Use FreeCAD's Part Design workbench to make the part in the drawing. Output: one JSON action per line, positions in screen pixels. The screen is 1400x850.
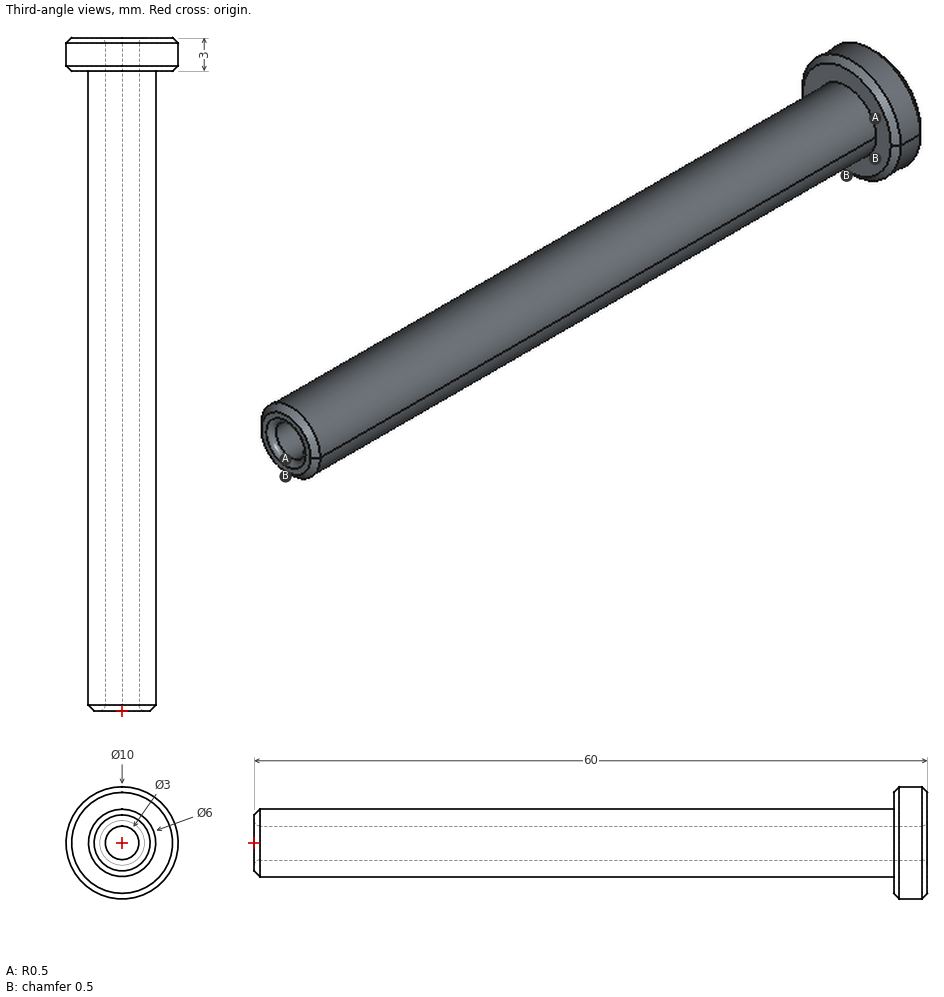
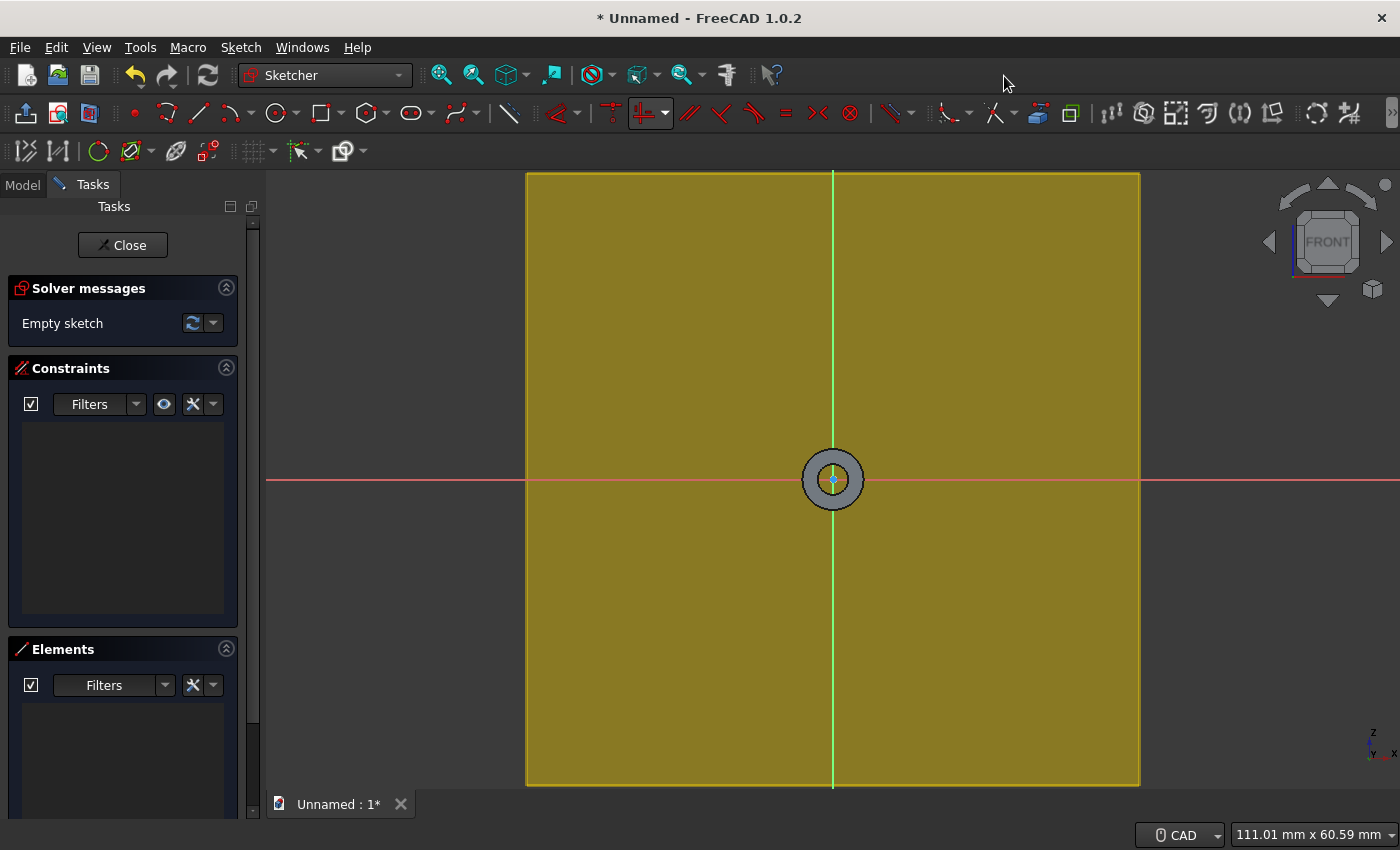
{"action": "left_click", "coordinate": [90, 114]}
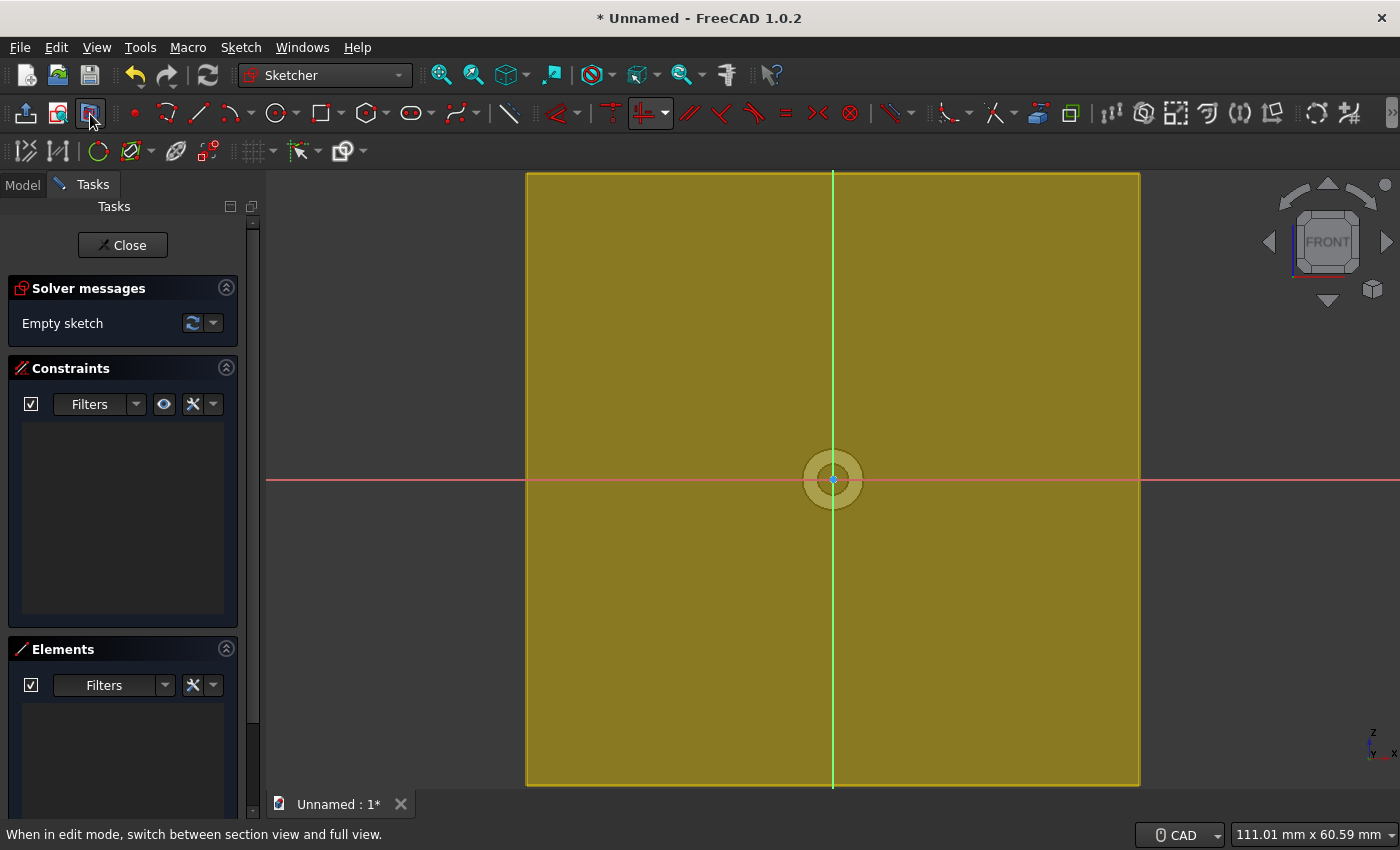
{"action": "scroll", "coordinate": [855, 480], "scroll_direction": "up", "scroll_amount": 7}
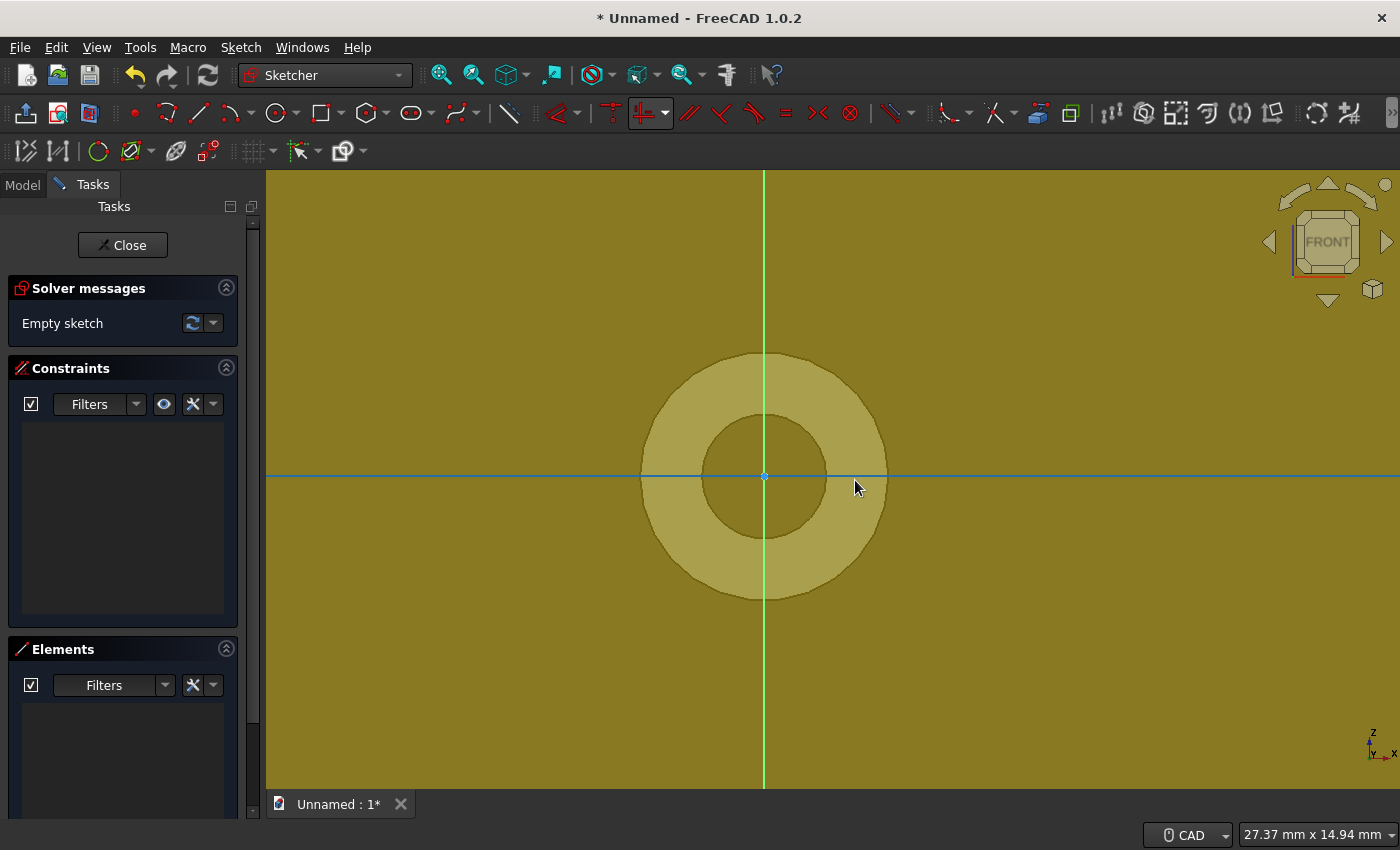
{"action": "key", "text": "g c"}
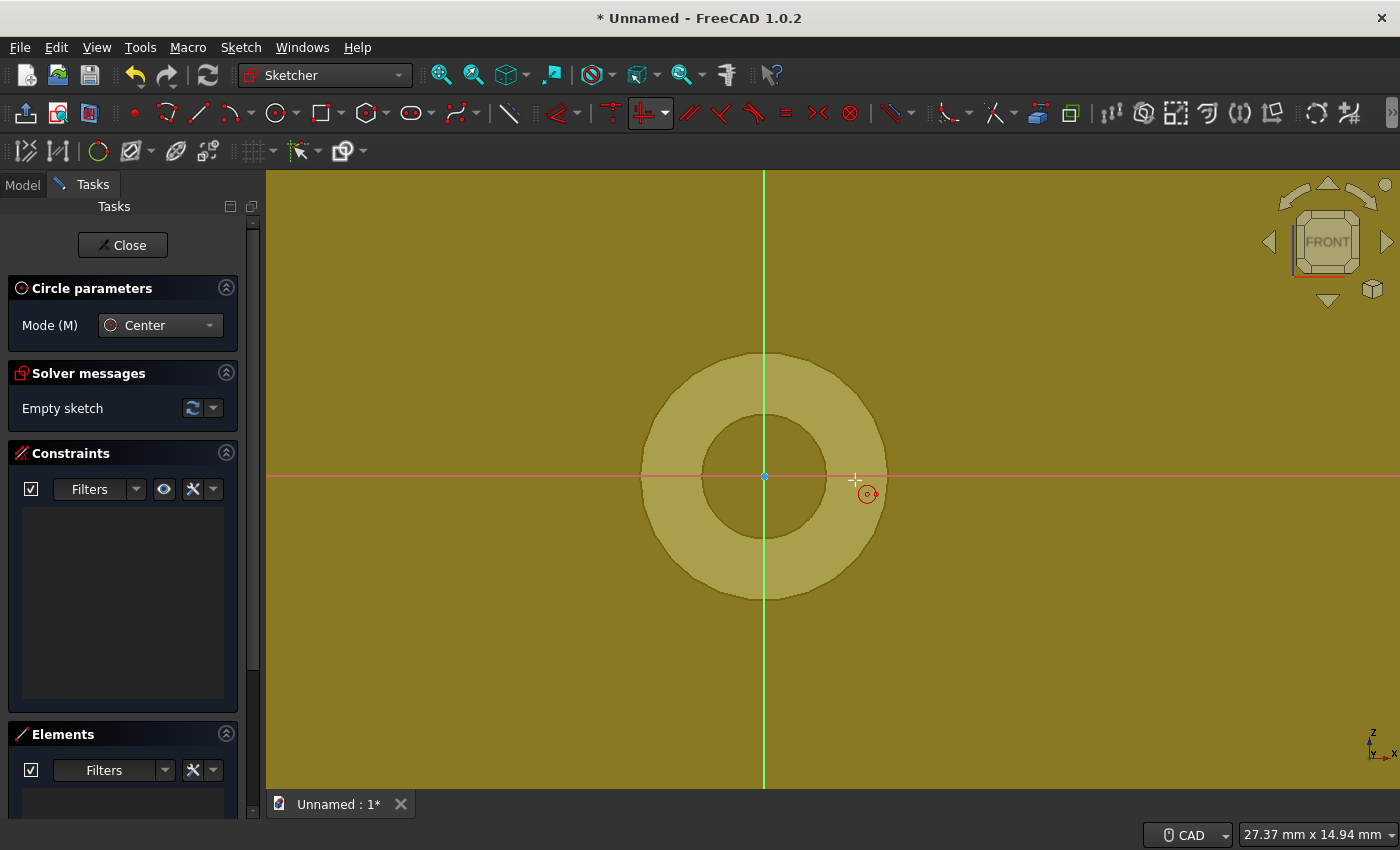
{"action": "left_click", "coordinate": [764, 476]}
{"action": "mouse_move", "coordinate": [911, 330]}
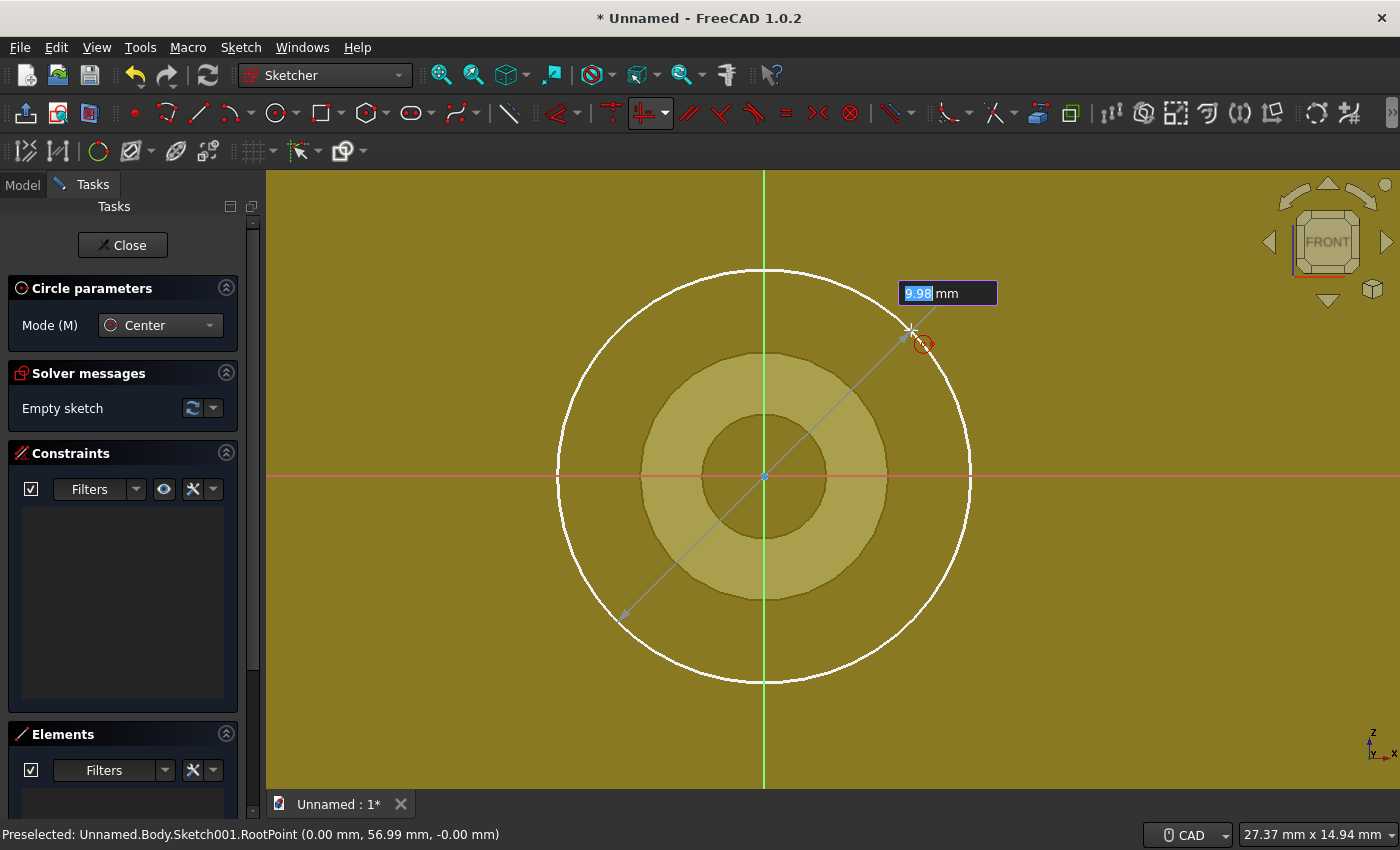
{"action": "type", "text": "10"}
{"action": "key", "text": "Return"}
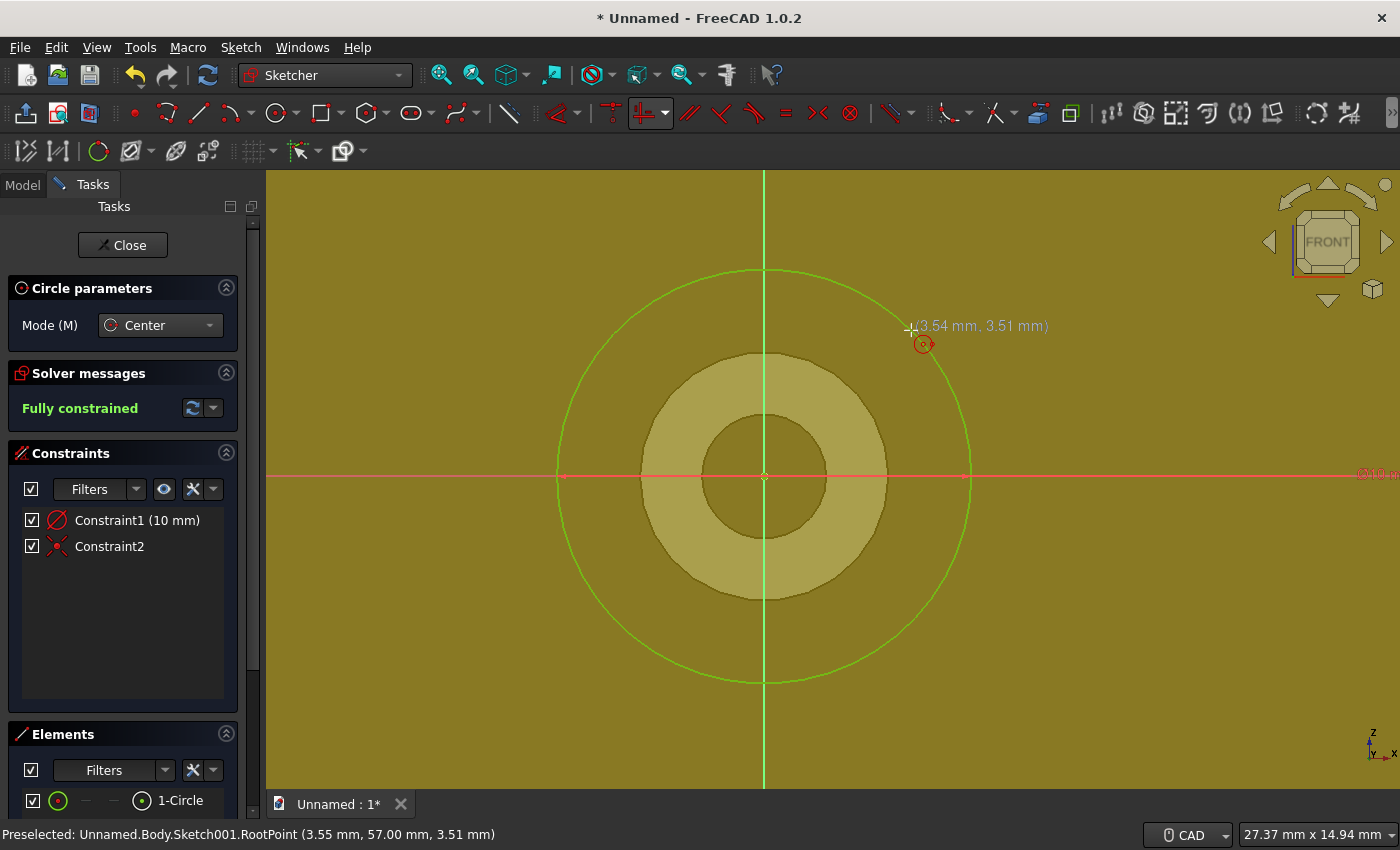
{"action": "left_click", "coordinate": [764, 476]}
{"action": "mouse_move", "coordinate": [808, 433]}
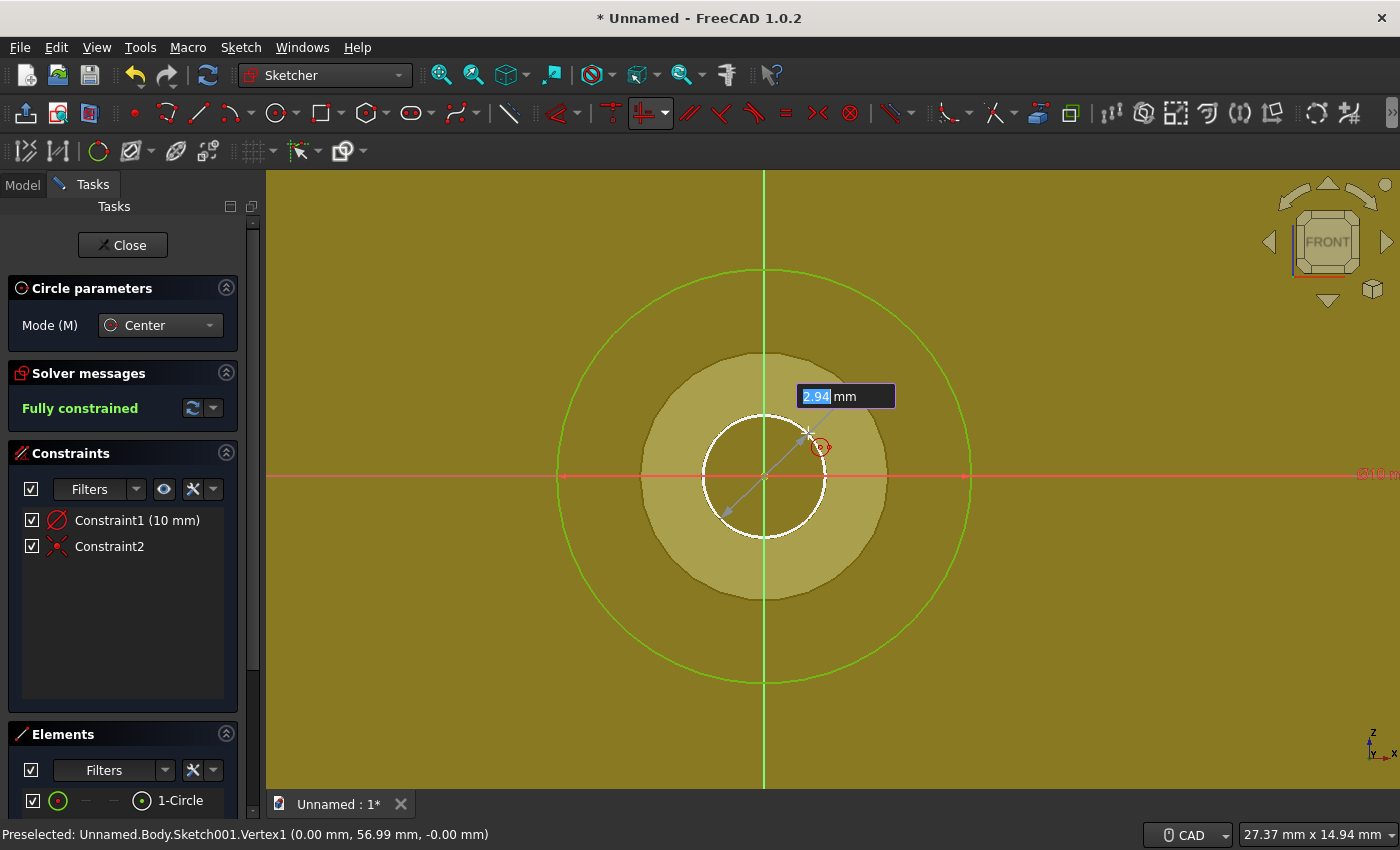
{"action": "type", "text": "3"}
{"action": "key", "text": "Return"}
{"action": "key", "text": "Escape"}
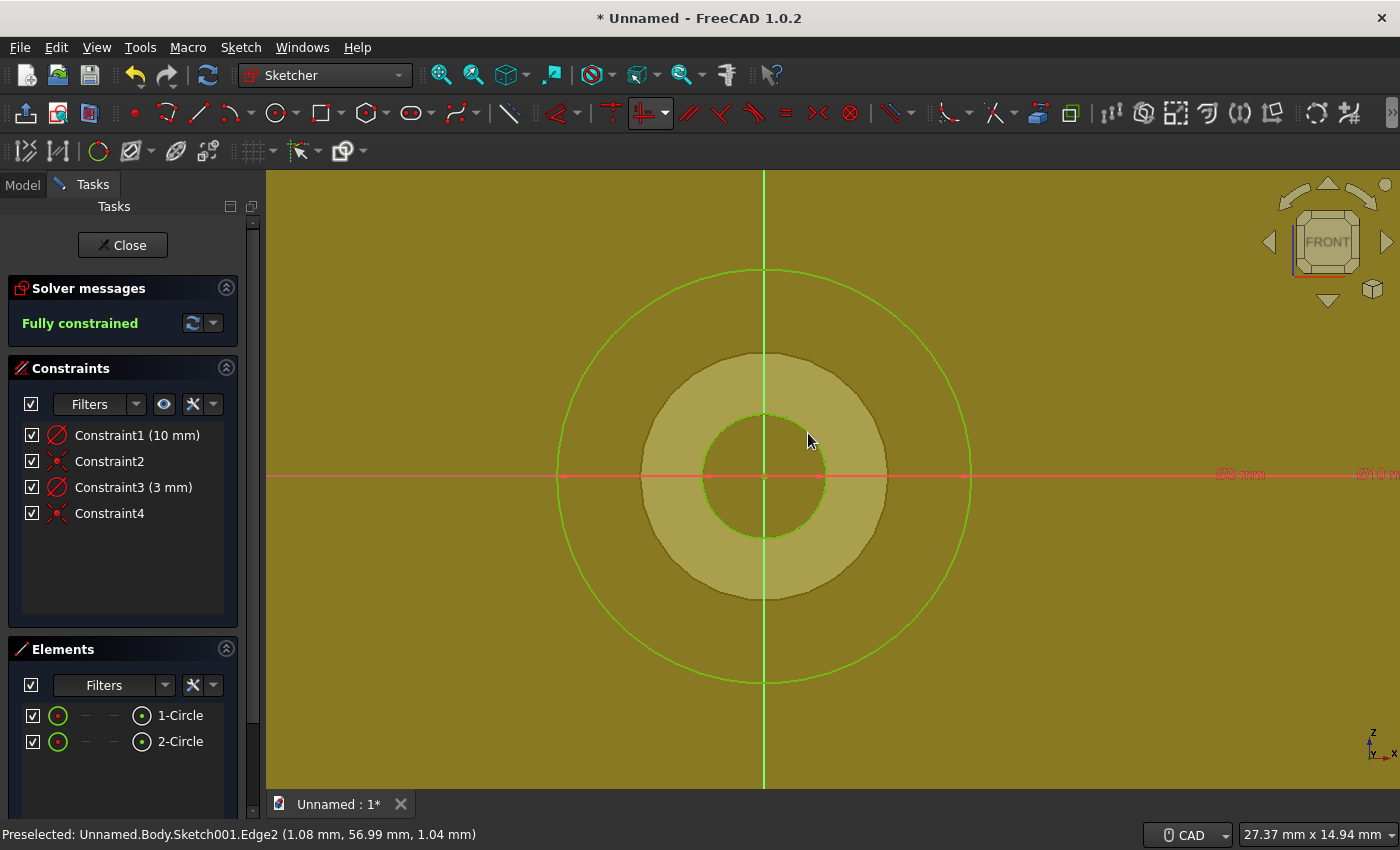
{"action": "left_click", "coordinate": [123, 245]}